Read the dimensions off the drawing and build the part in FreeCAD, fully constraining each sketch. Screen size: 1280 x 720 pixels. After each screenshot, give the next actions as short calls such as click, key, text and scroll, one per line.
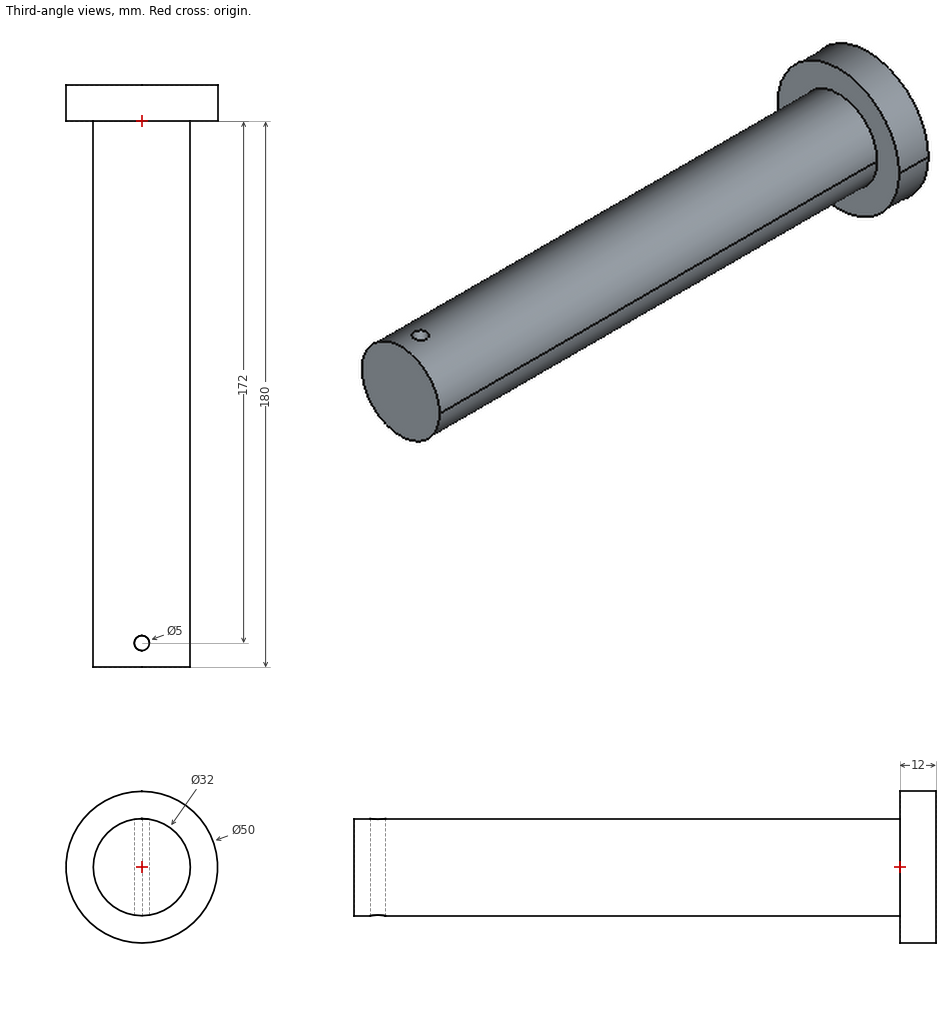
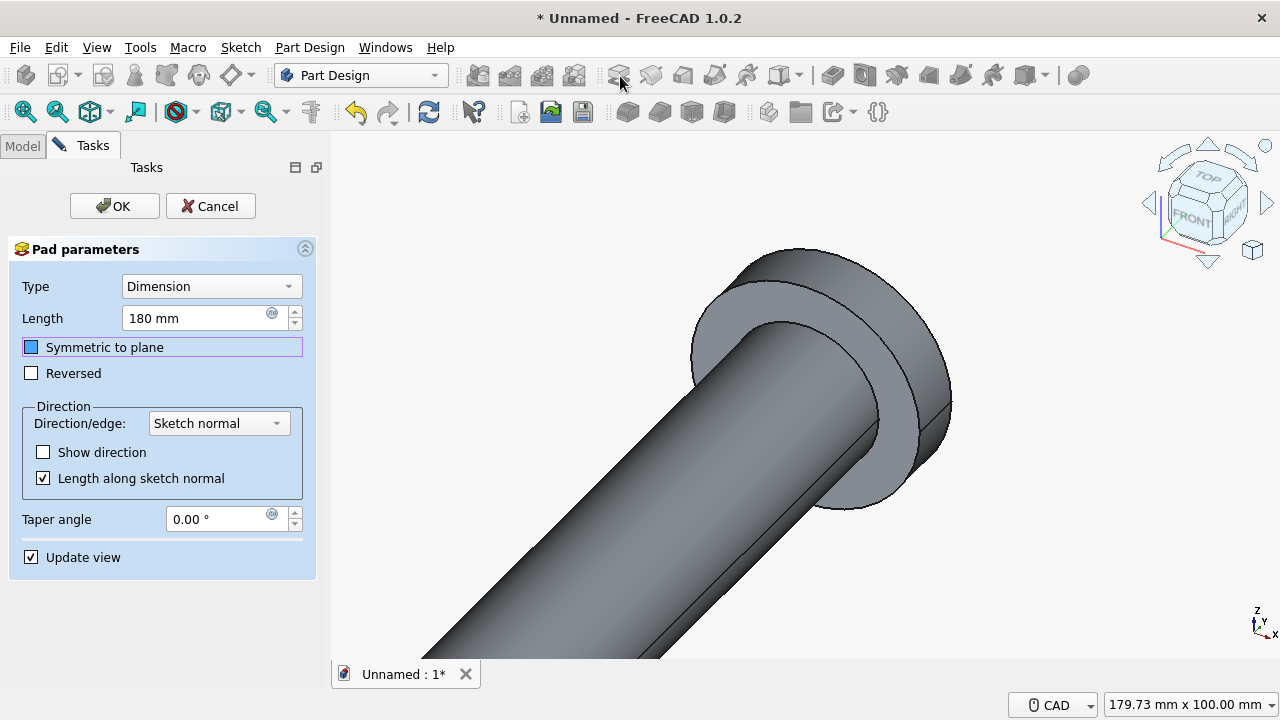
click(115, 206)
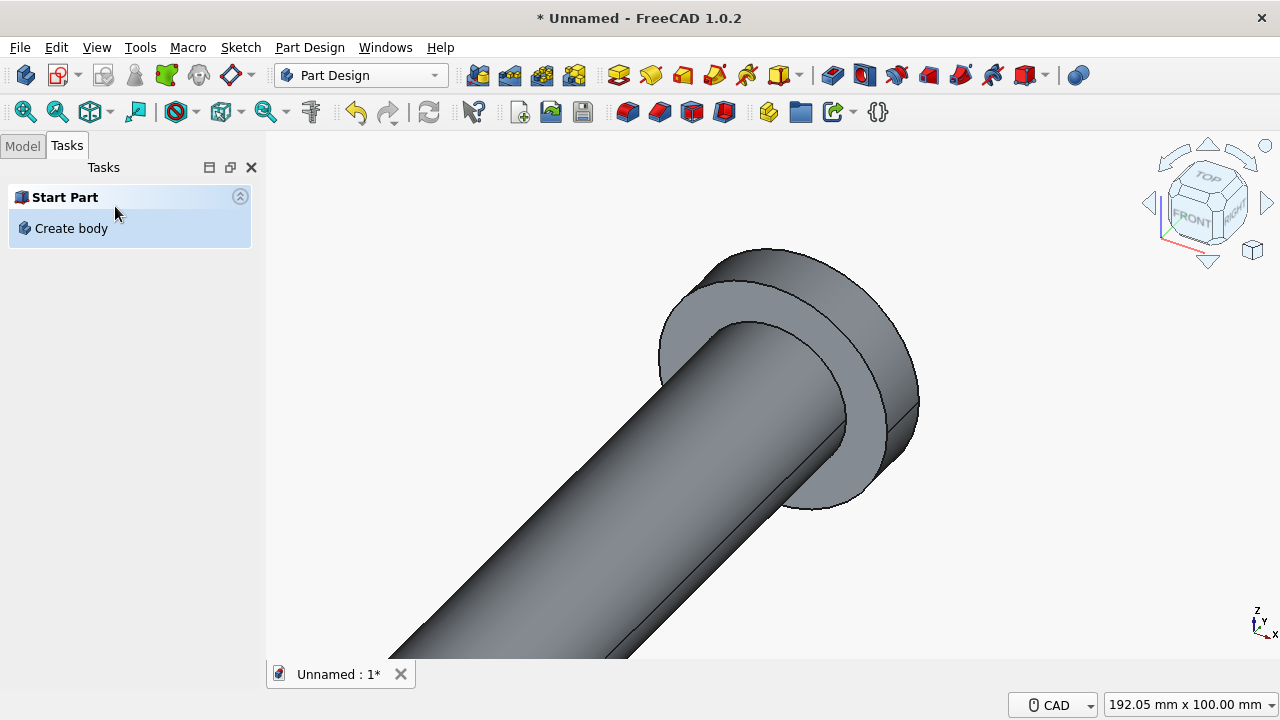
click(26, 112)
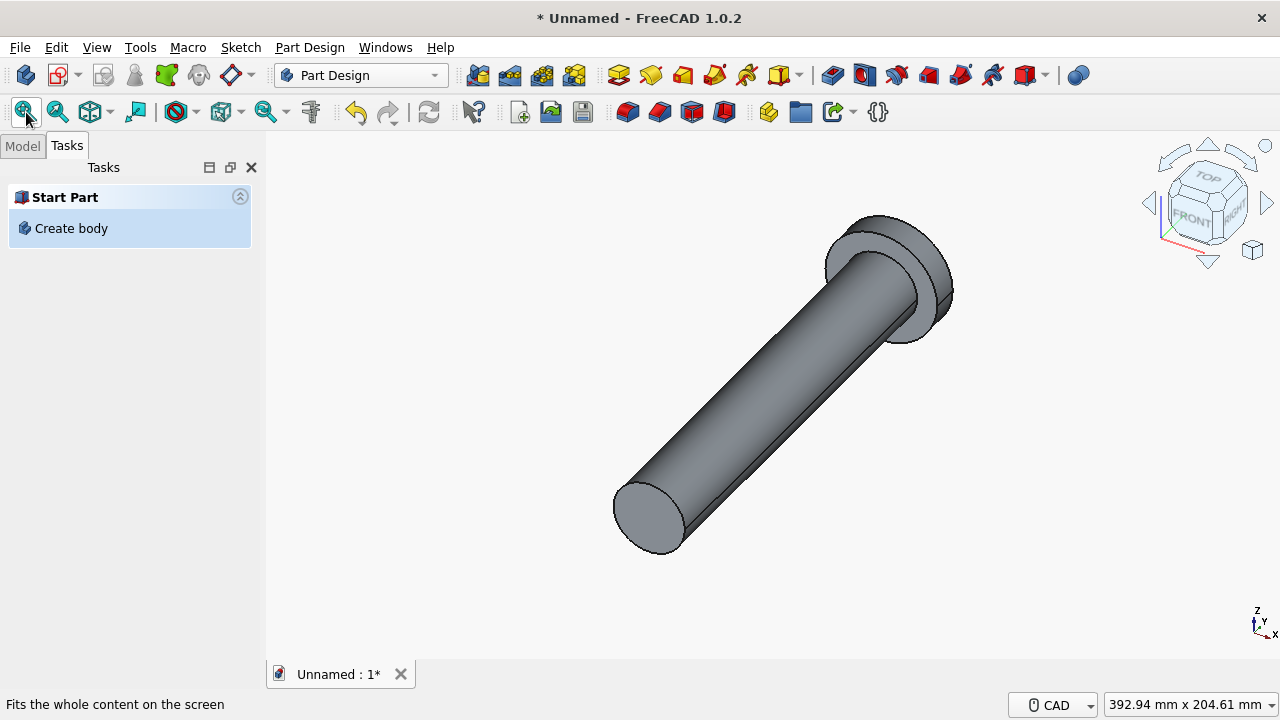
click(58, 76)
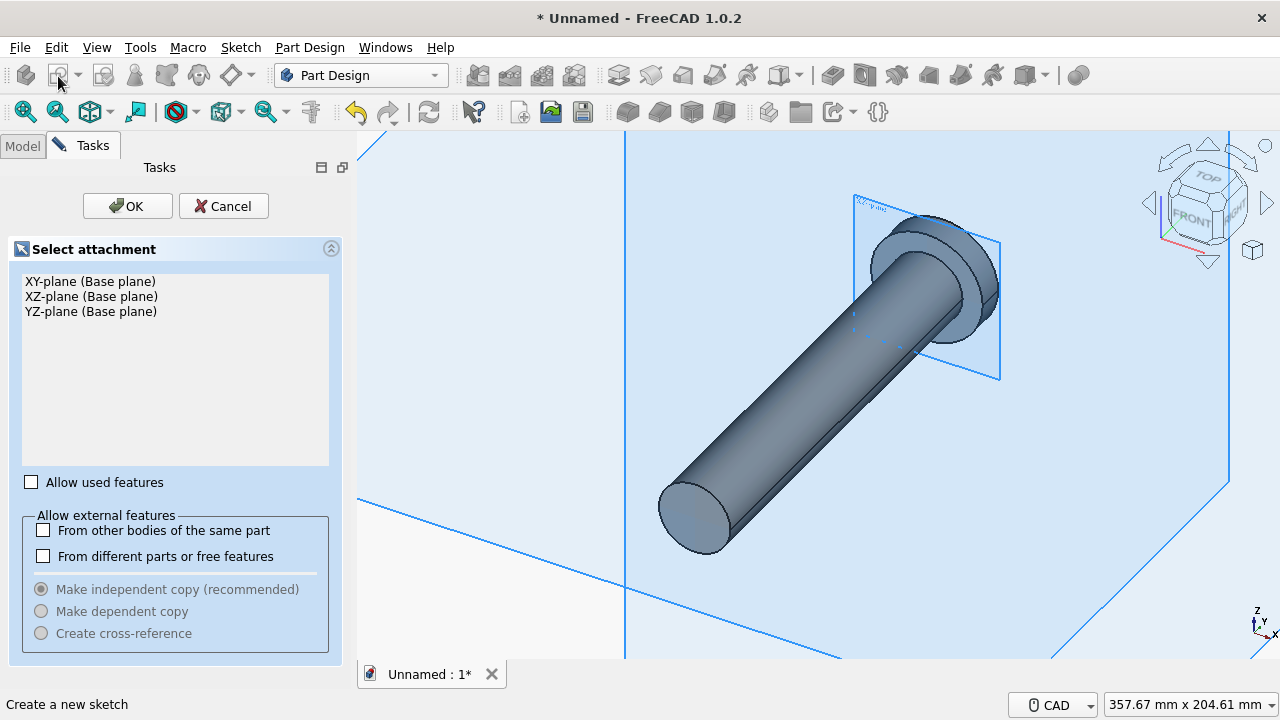
click(82, 282)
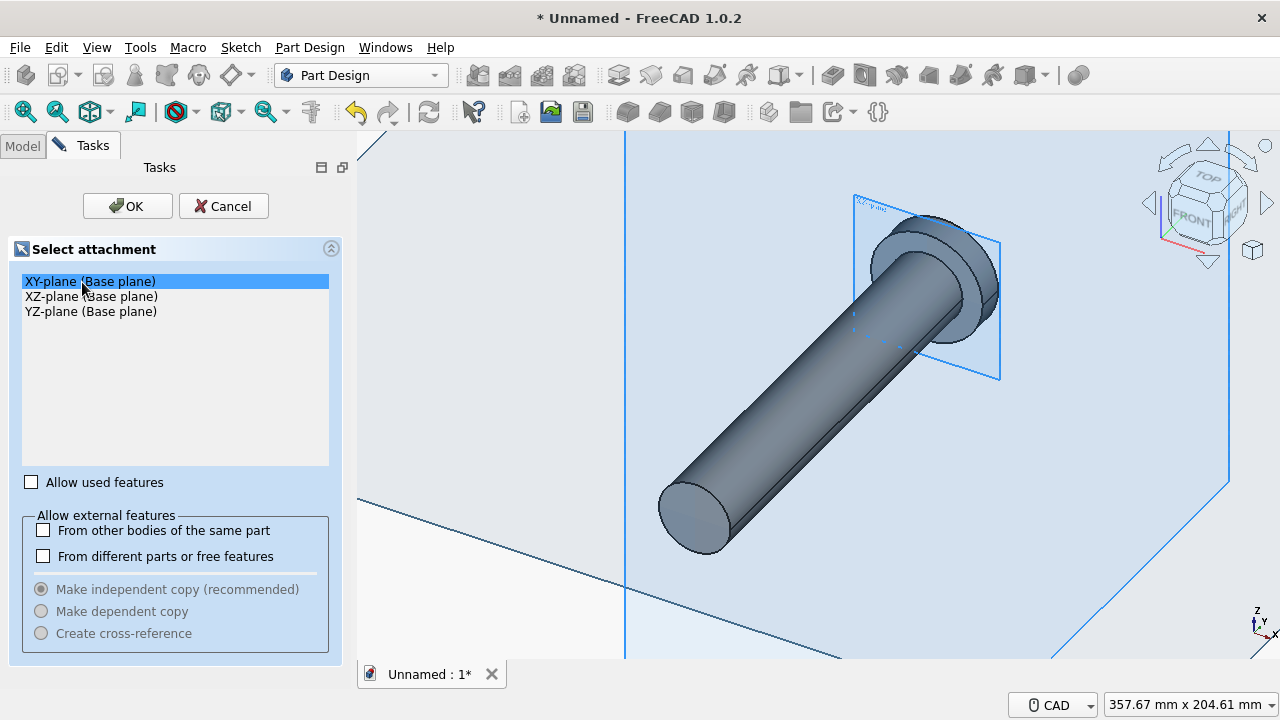
click(128, 206)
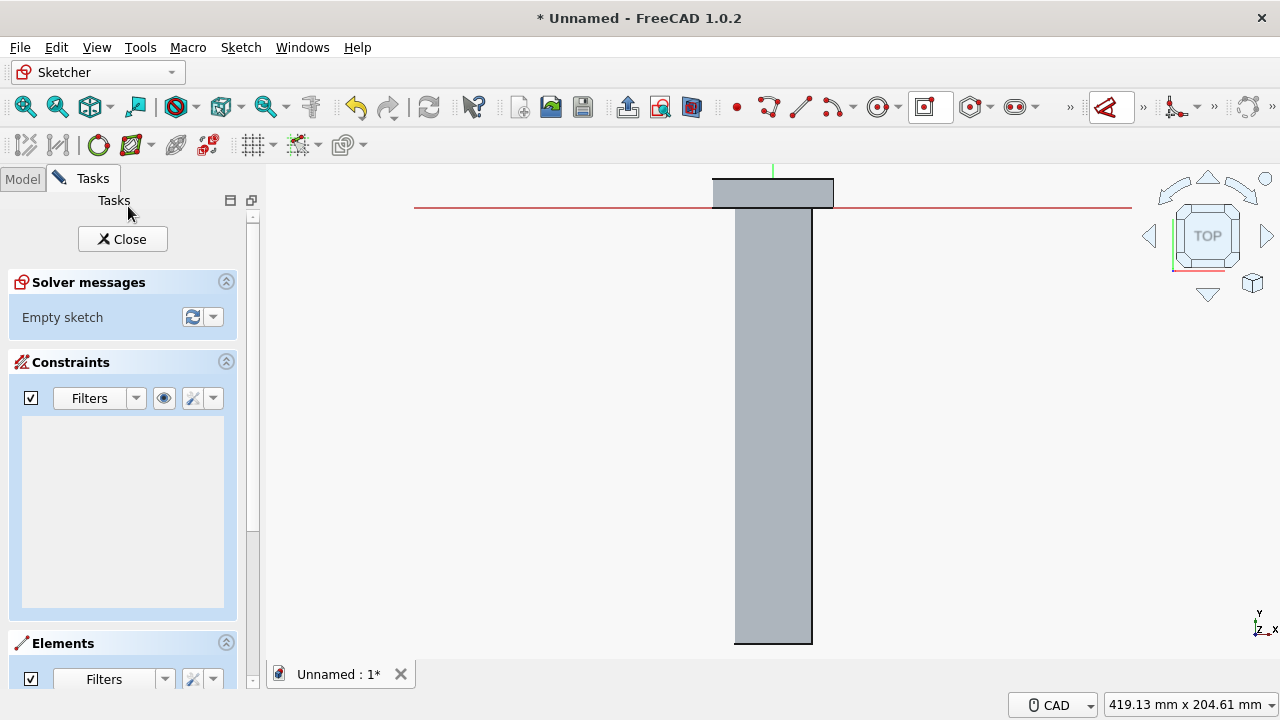
click(692, 108)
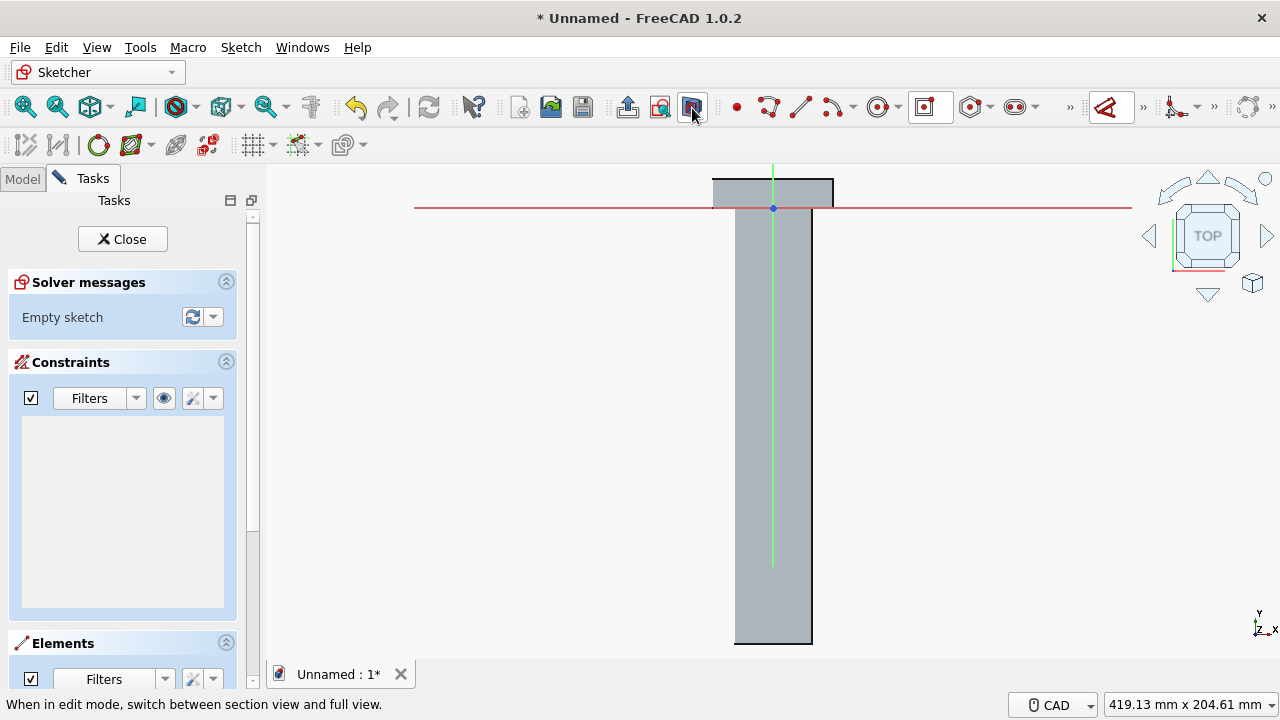
scroll(704, 412, down, 5)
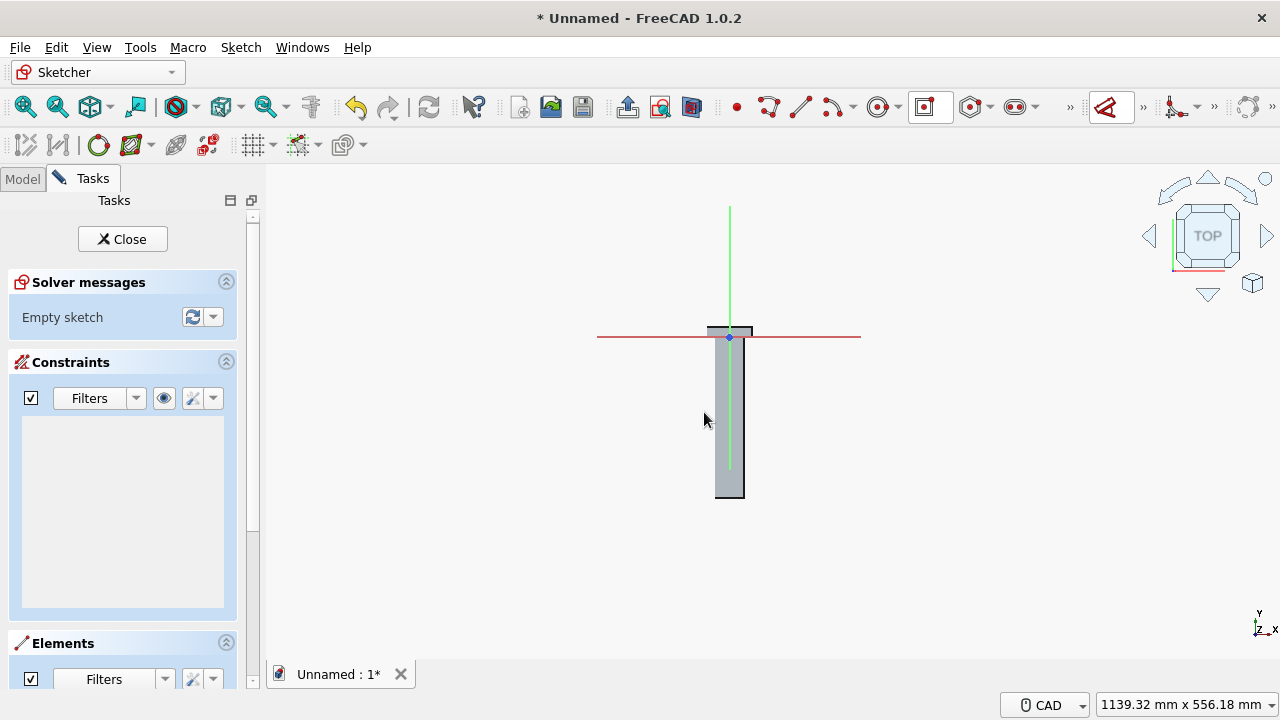
scroll(731, 495, up, 15)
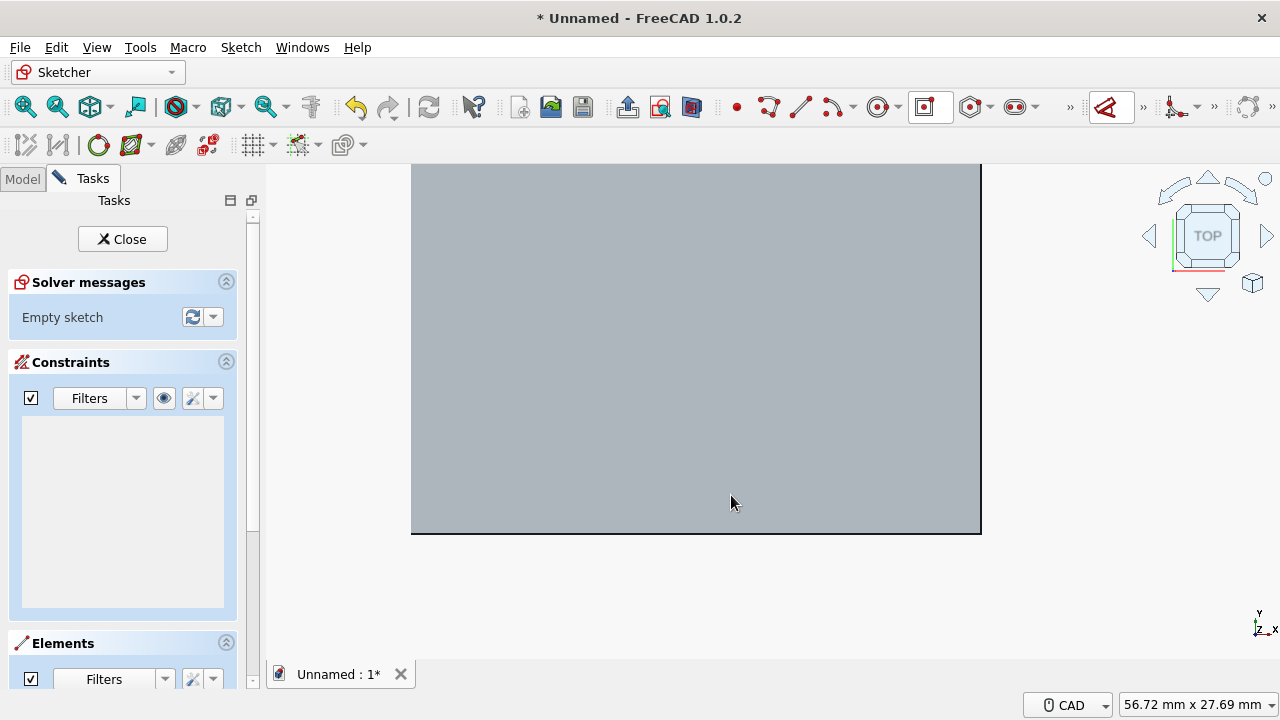
scroll(691, 382, up, 6)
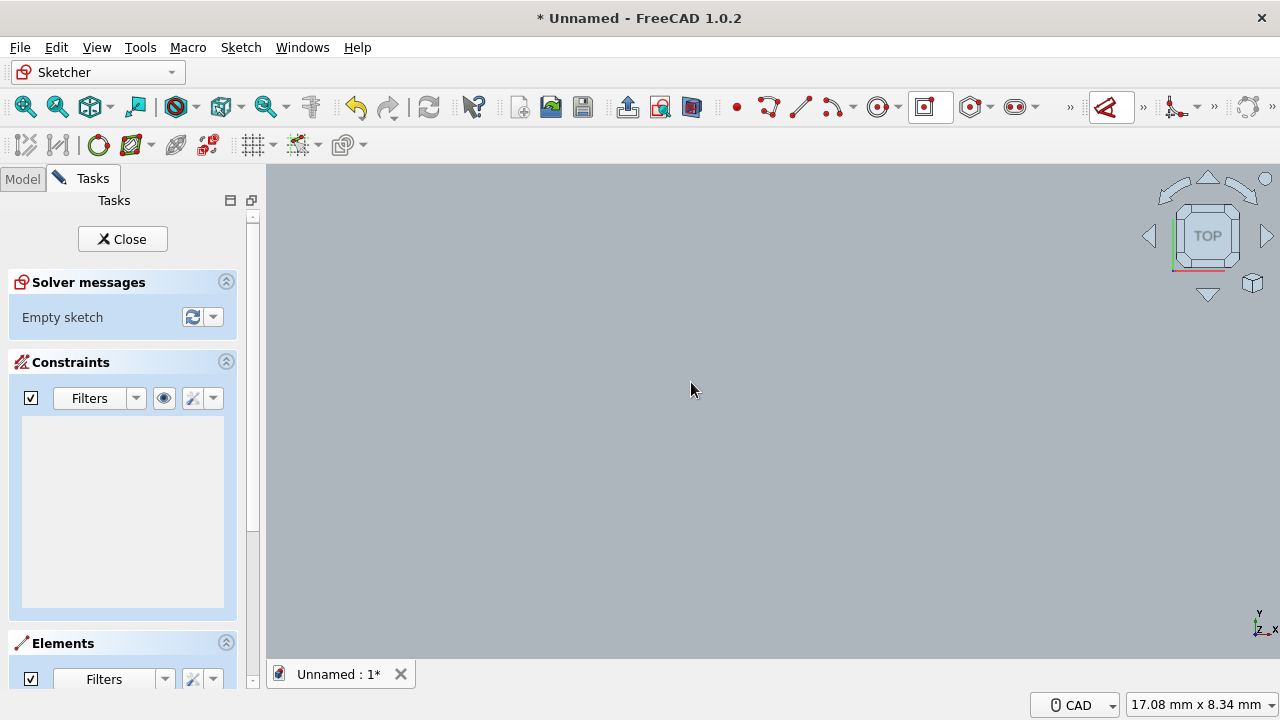
click(878, 108)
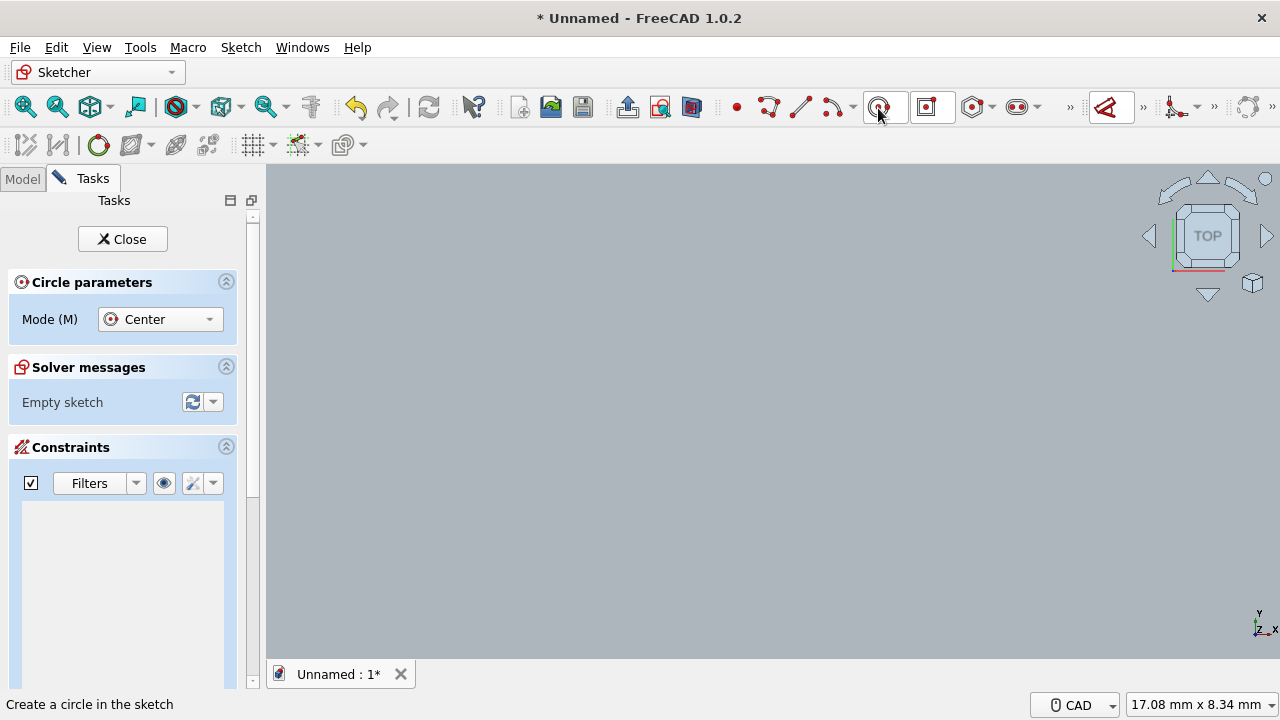
click(704, 410)
move(809, 306)